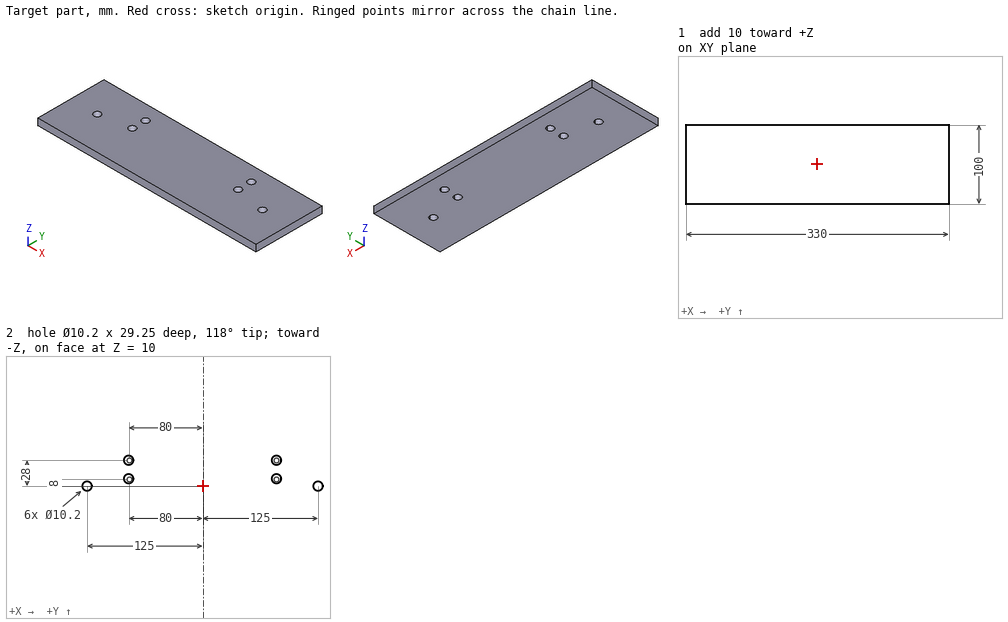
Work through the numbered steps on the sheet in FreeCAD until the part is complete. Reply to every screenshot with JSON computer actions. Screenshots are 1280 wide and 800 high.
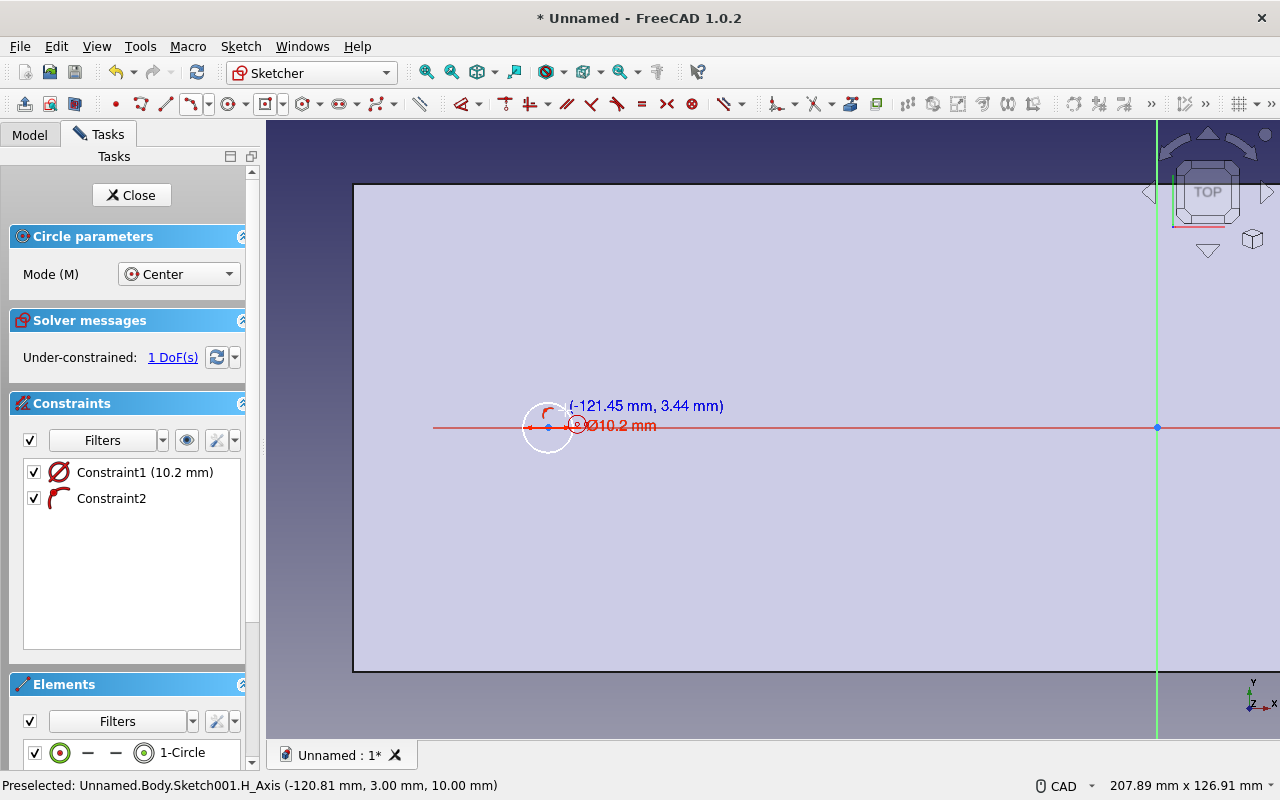
{"action": "left_click", "coordinate": [767, 389]}
{"action": "mouse_move", "coordinate": [785, 371]}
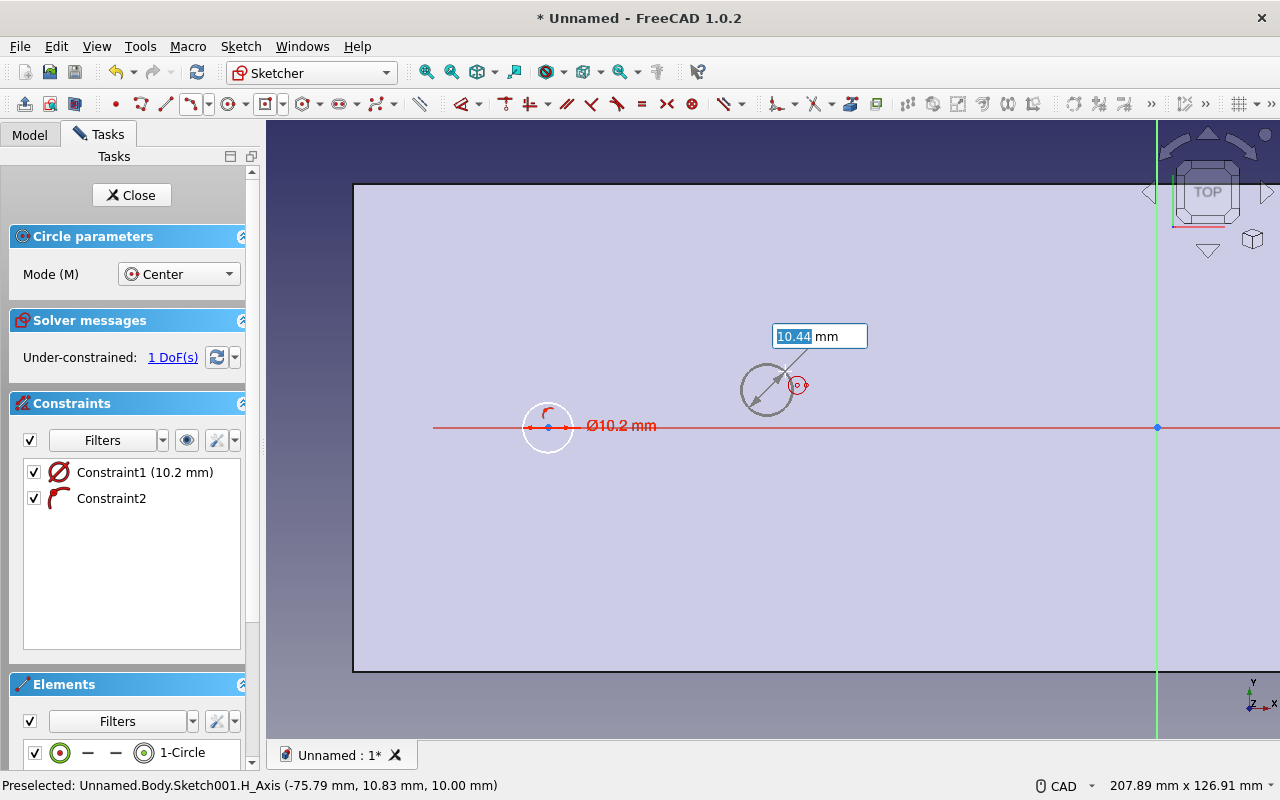
{"action": "type", "text": "10.2"}
{"action": "key", "text": "Return"}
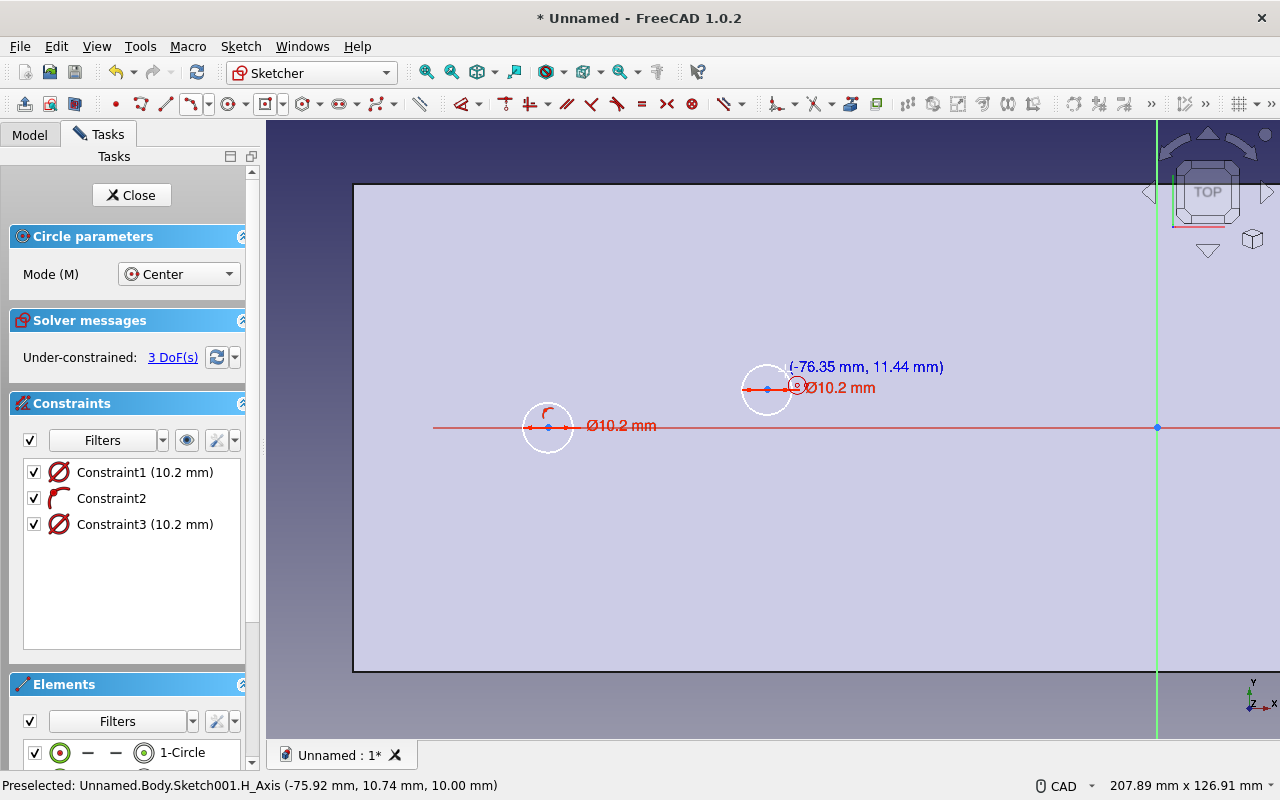
{"action": "left_click", "coordinate": [767, 291]}
{"action": "mouse_move", "coordinate": [785, 274]}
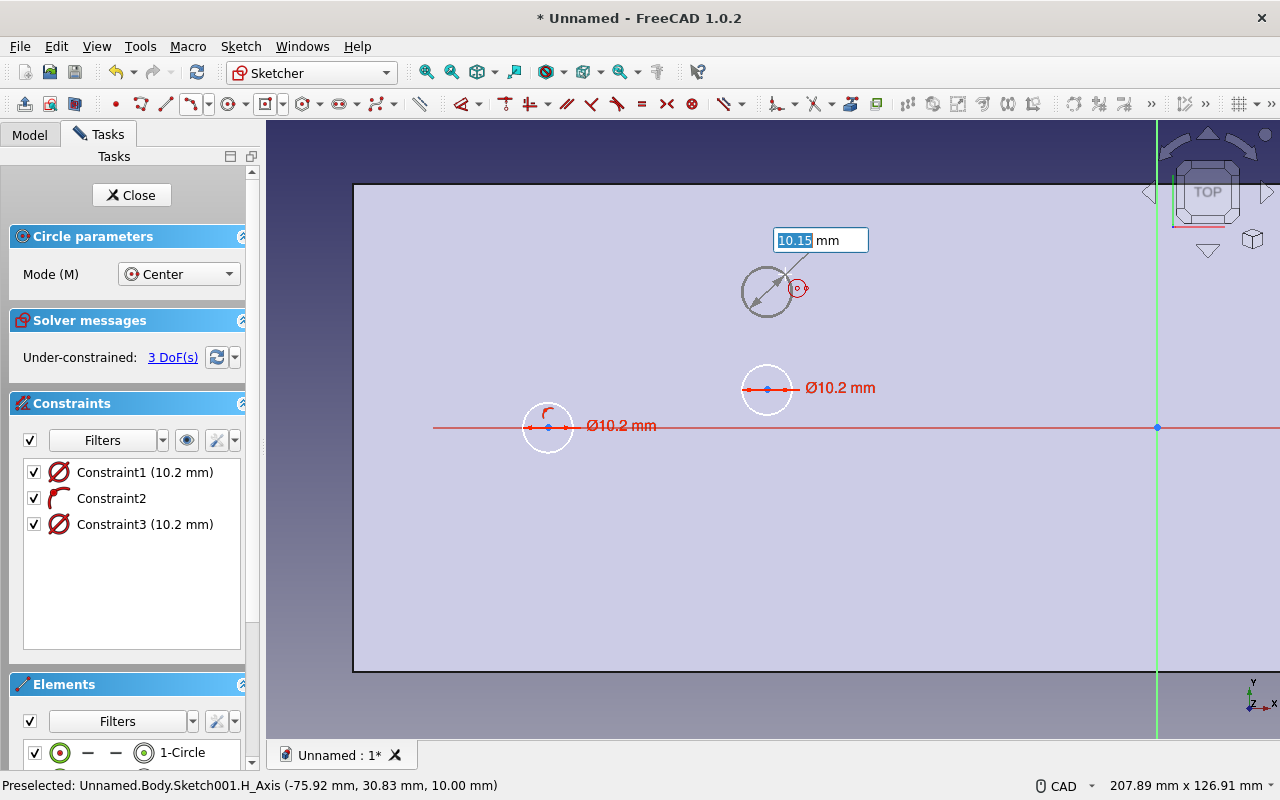
{"action": "type", "text": "10.2"}
{"action": "key", "text": "Return"}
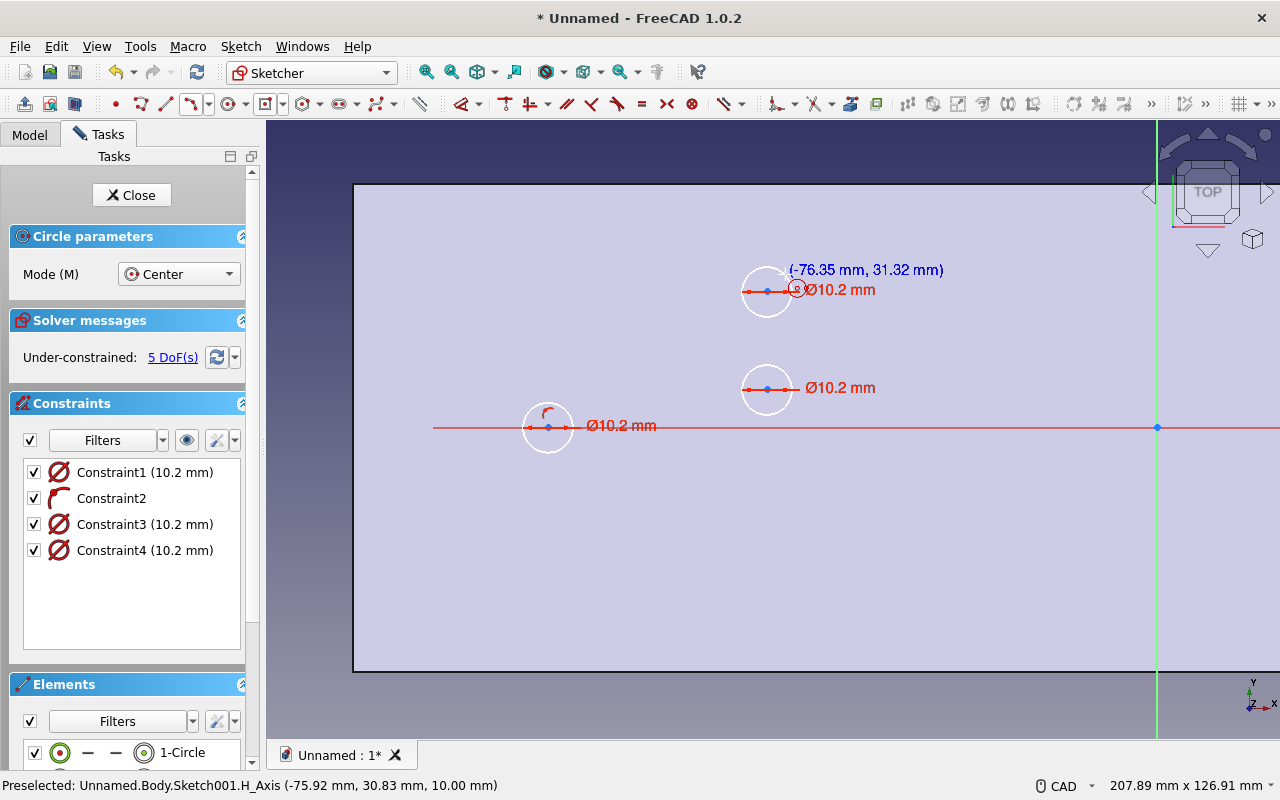
{"action": "scroll", "coordinate": [335, 487], "scroll_direction": "down", "scroll_amount": 4}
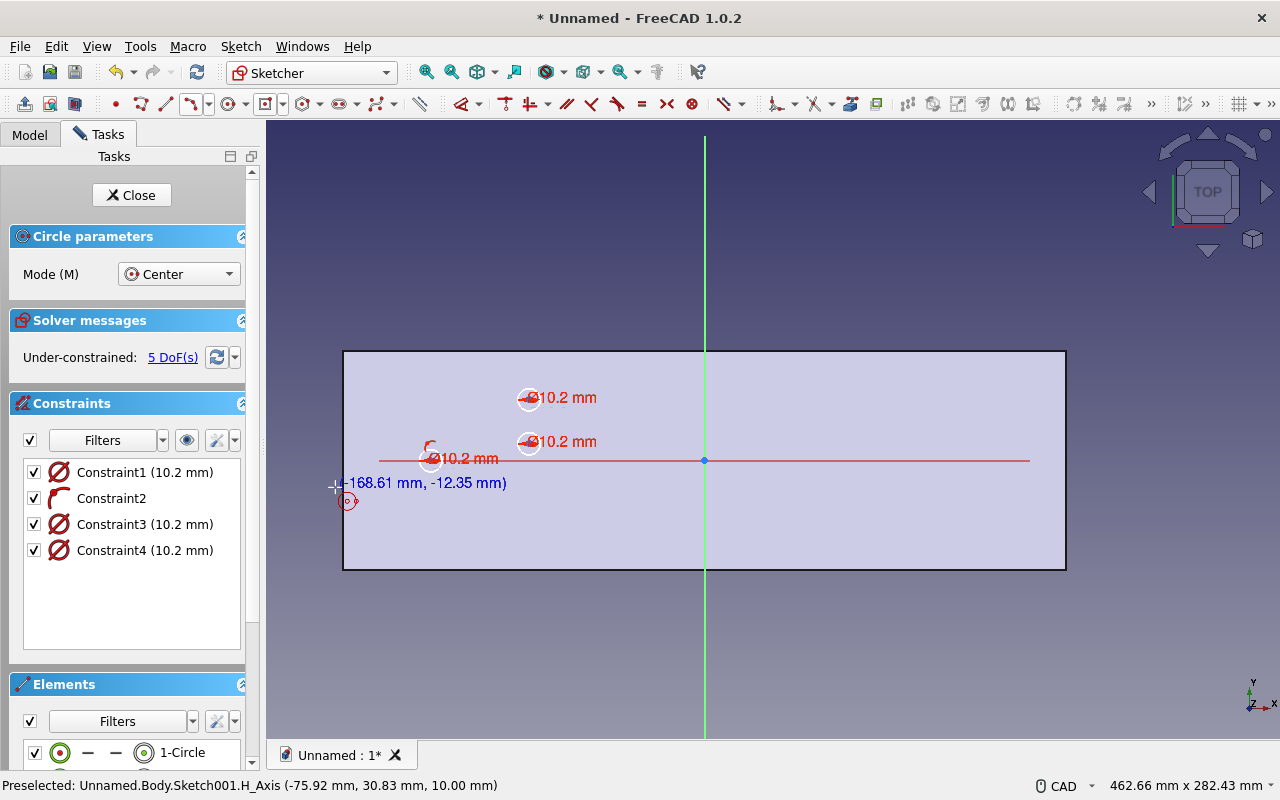
{"action": "scroll", "coordinate": [880, 399], "scroll_direction": "up", "scroll_amount": 4}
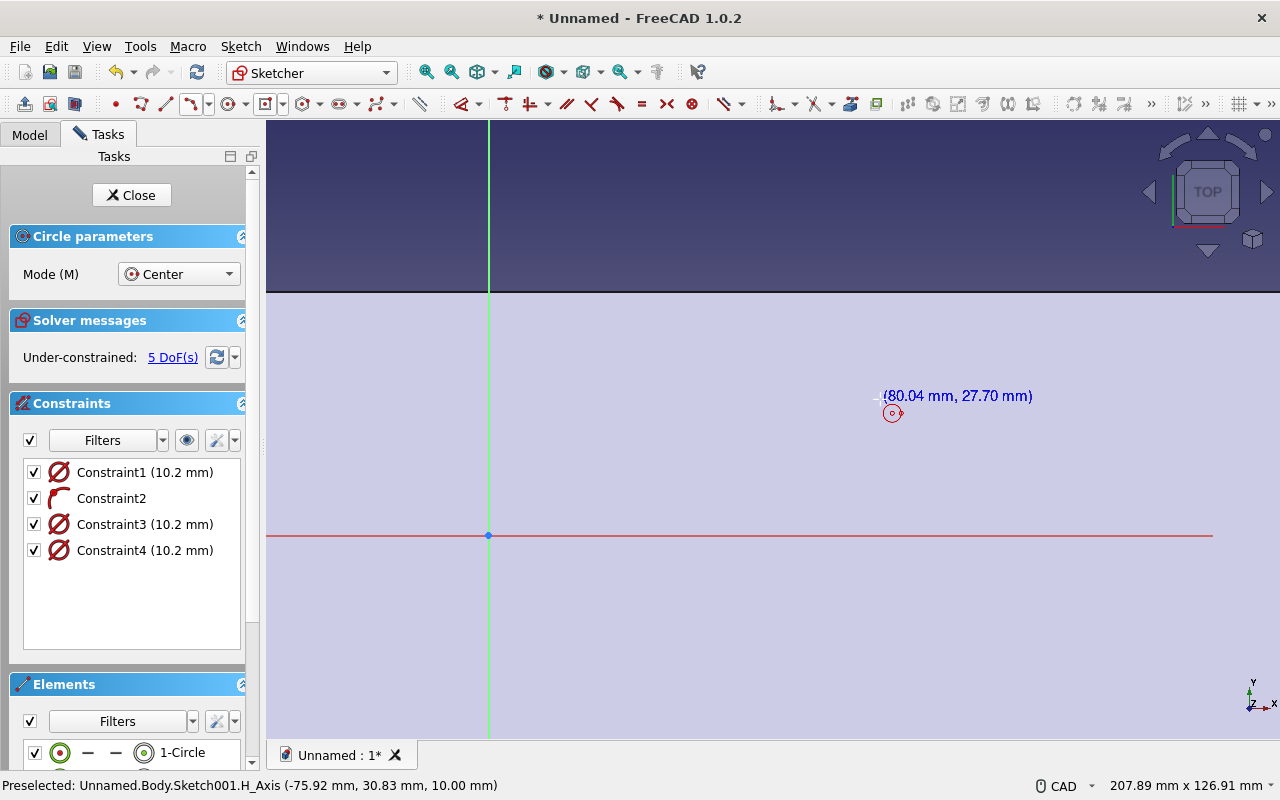
{"action": "left_click", "coordinate": [879, 399]}
{"action": "mouse_move", "coordinate": [897, 382]}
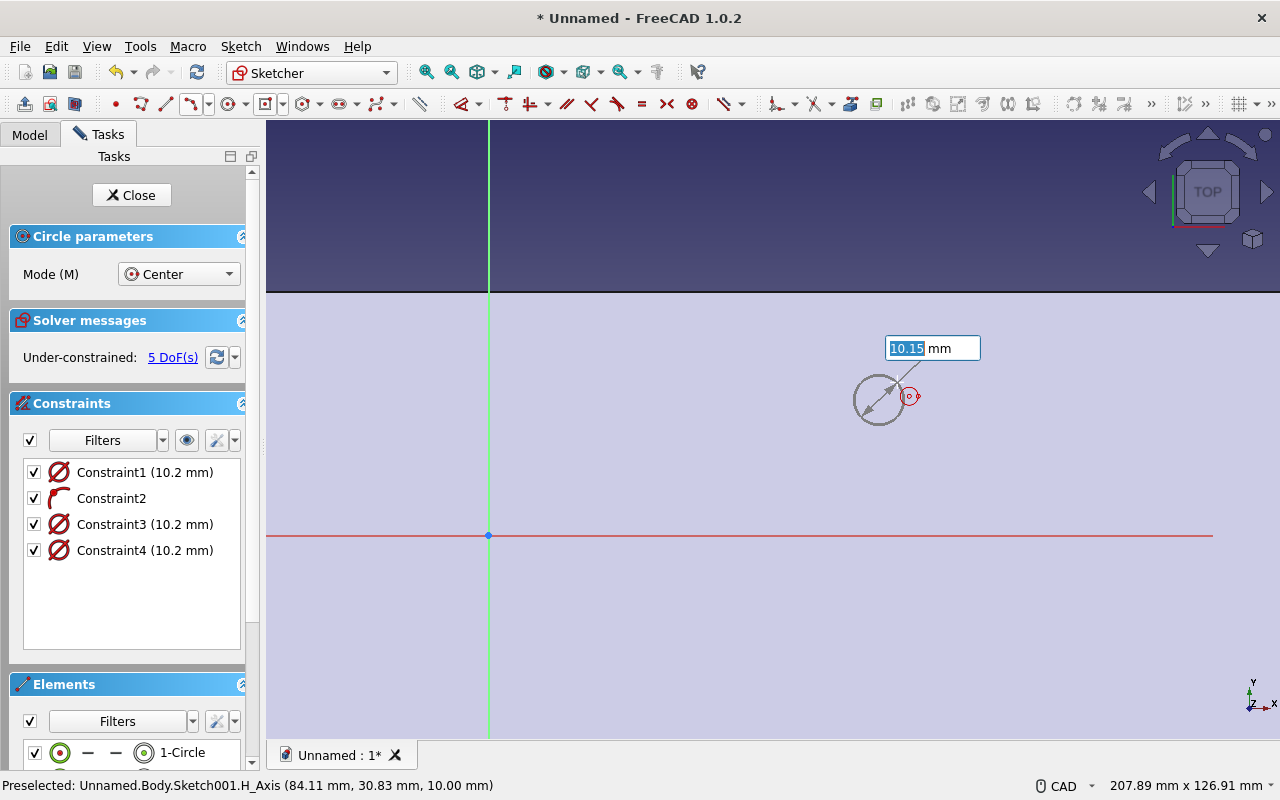
{"action": "type", "text": "10.2"}
{"action": "key", "text": "Return"}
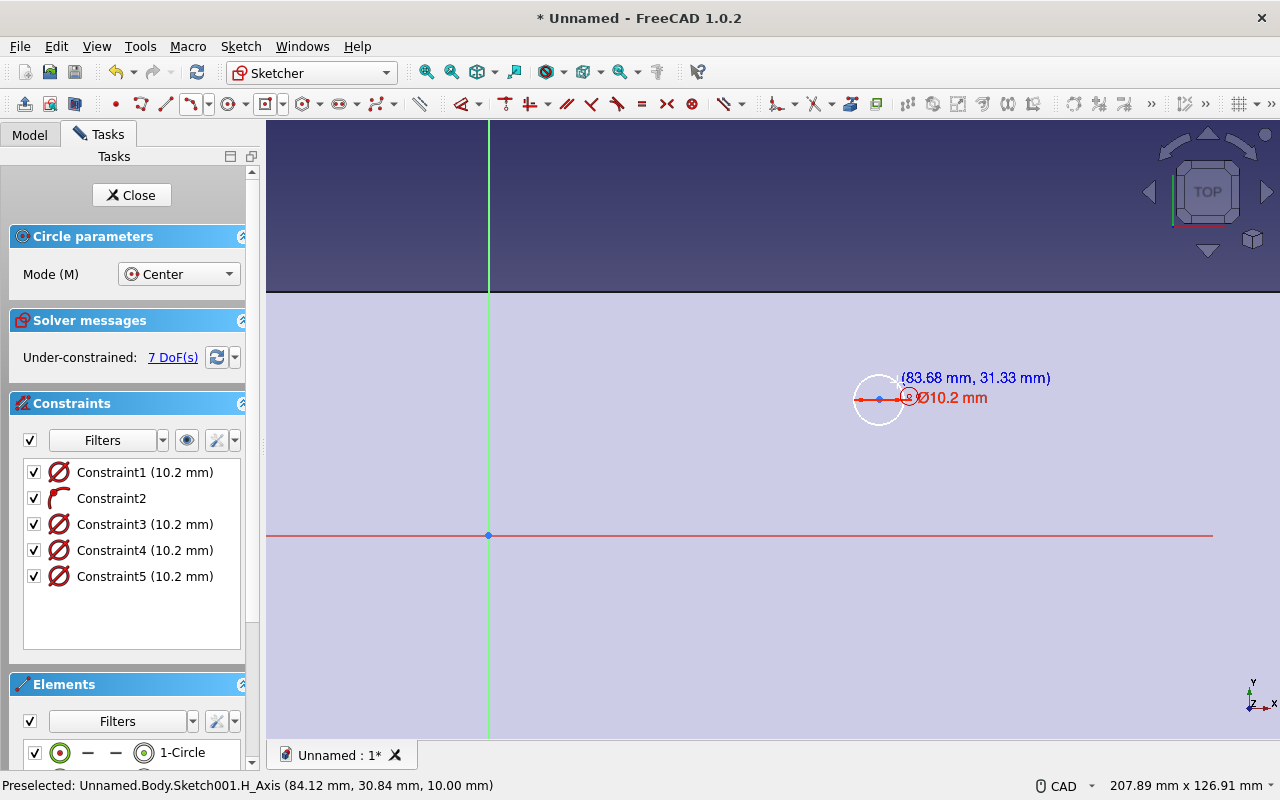
{"action": "left_click", "coordinate": [879, 497]}
{"action": "mouse_move", "coordinate": [897, 479]}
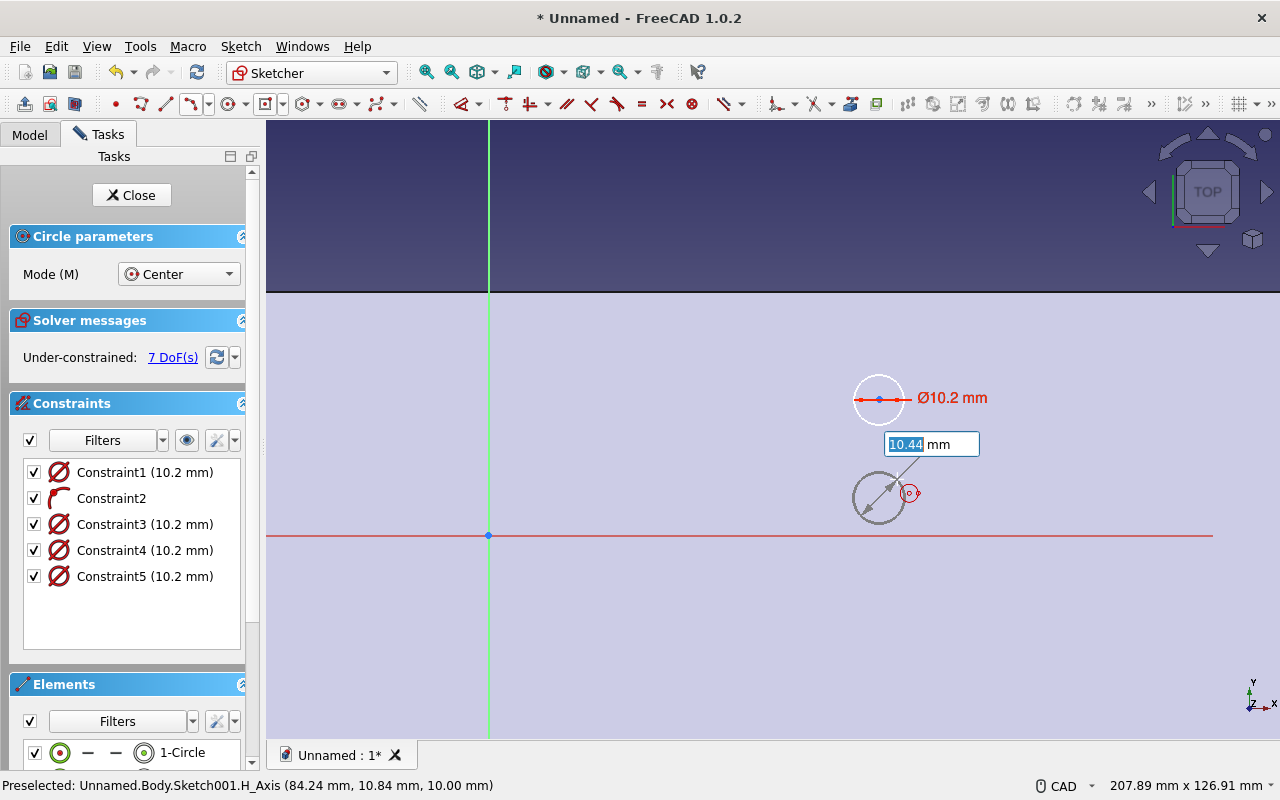
{"action": "type", "text": "10.2"}
{"action": "key", "text": "Return"}